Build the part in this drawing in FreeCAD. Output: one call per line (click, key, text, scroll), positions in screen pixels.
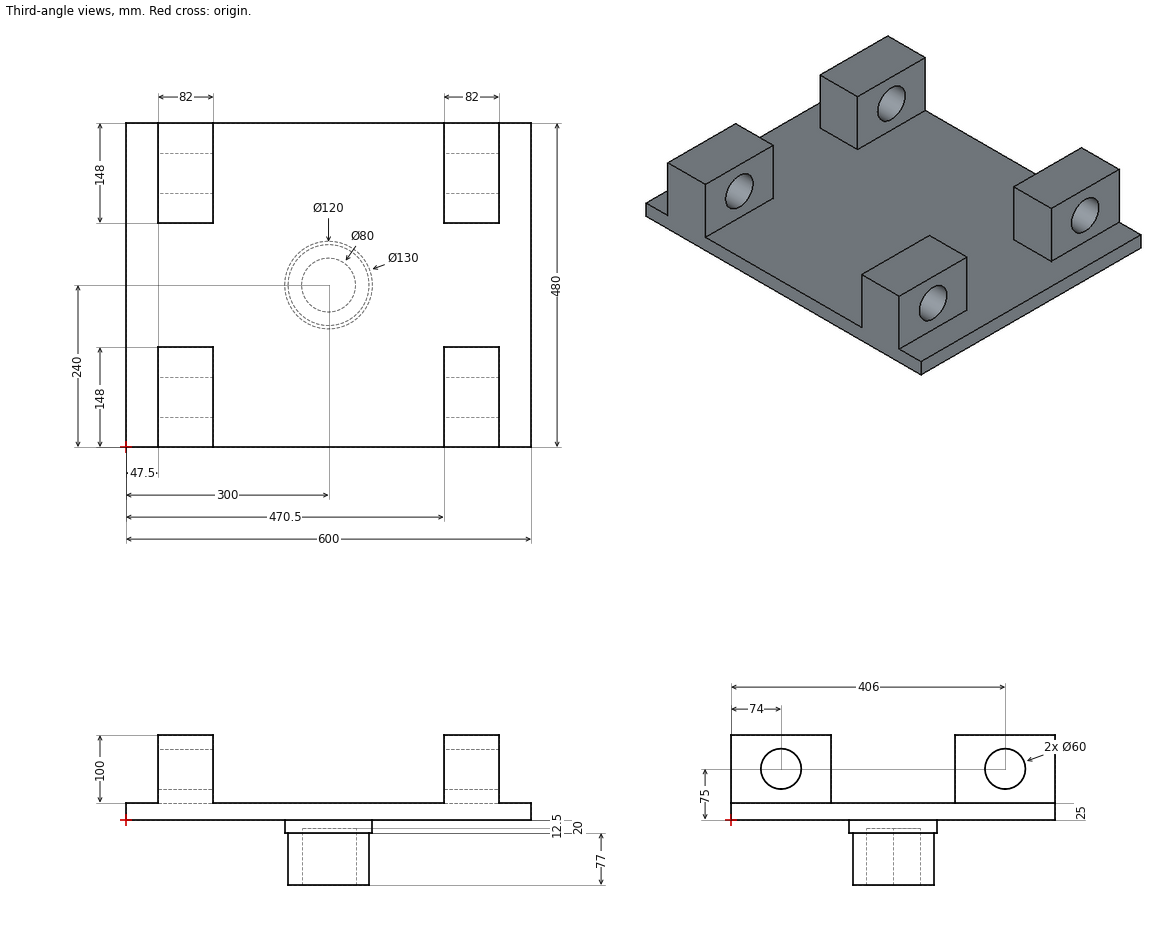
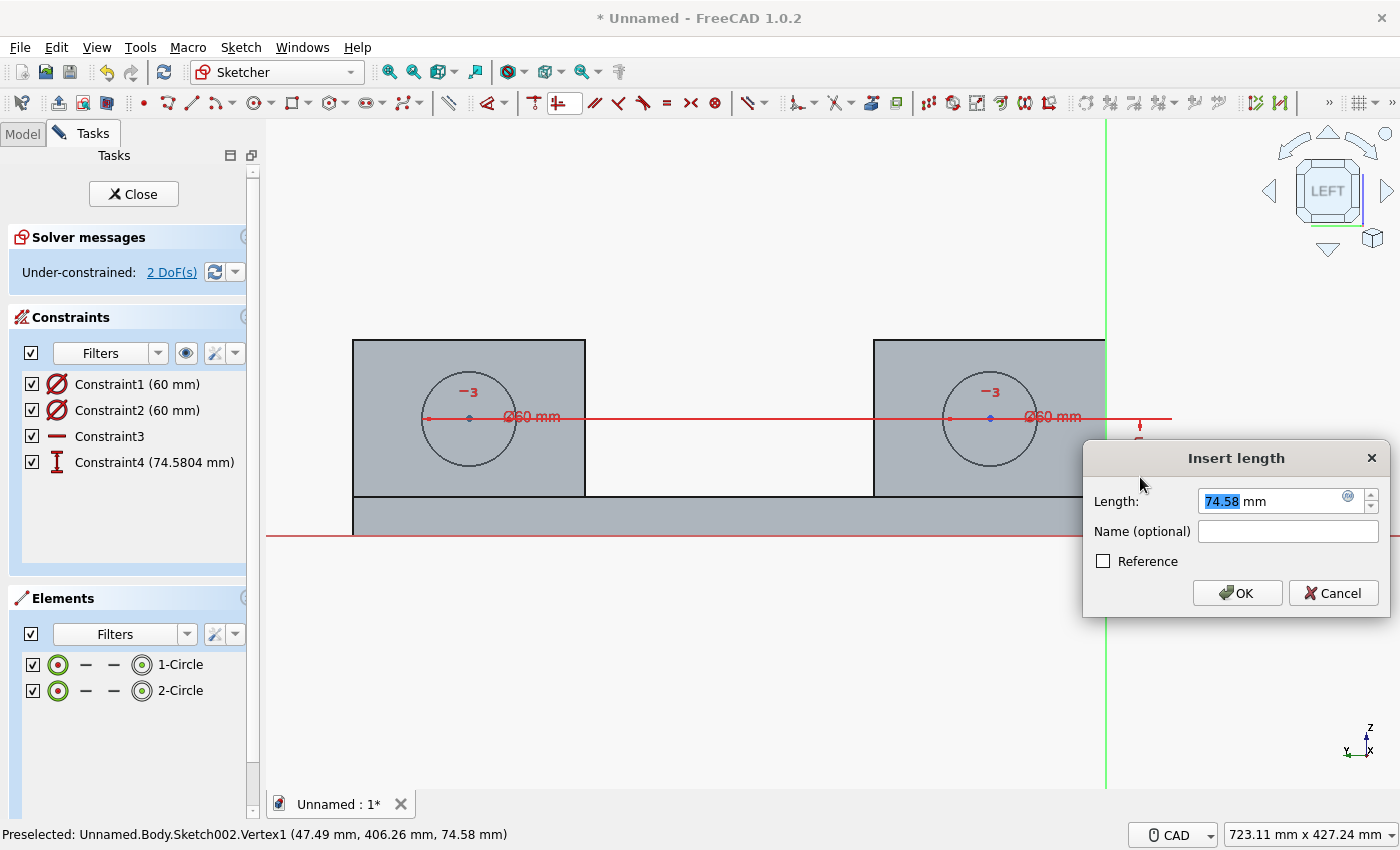
text(75)
key(Return)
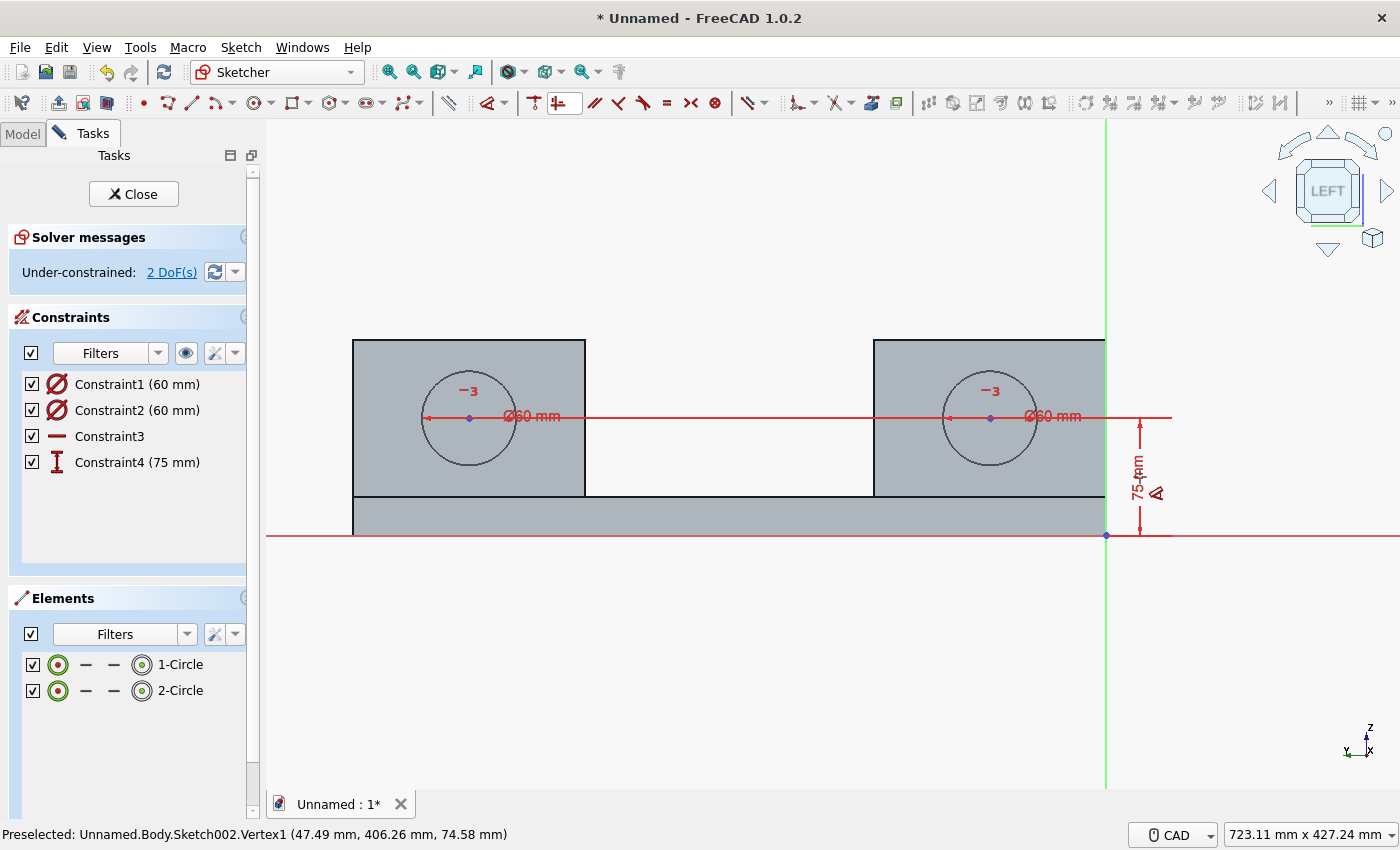
click(990, 418)
click(1048, 570)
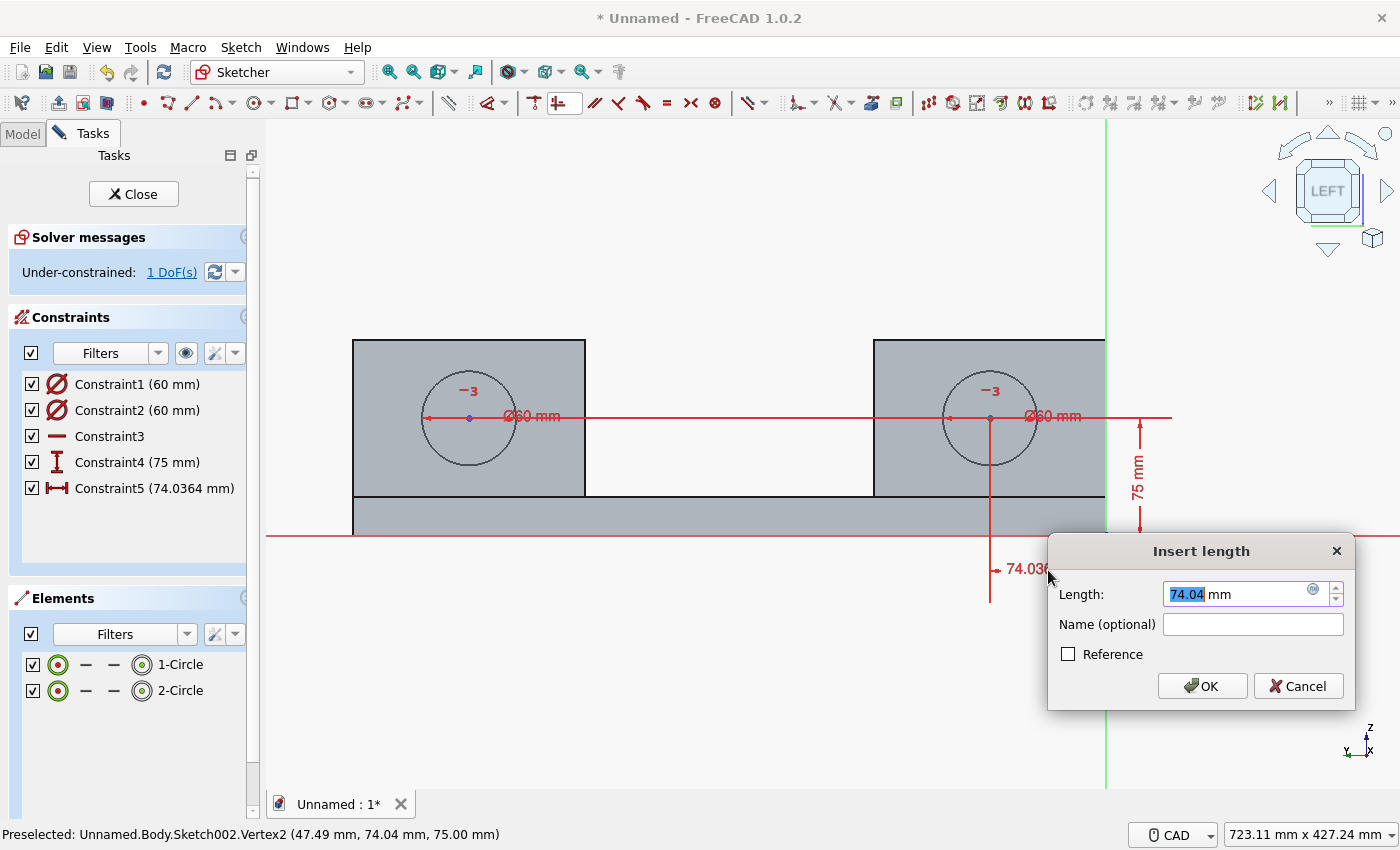
text(74)
key(Return)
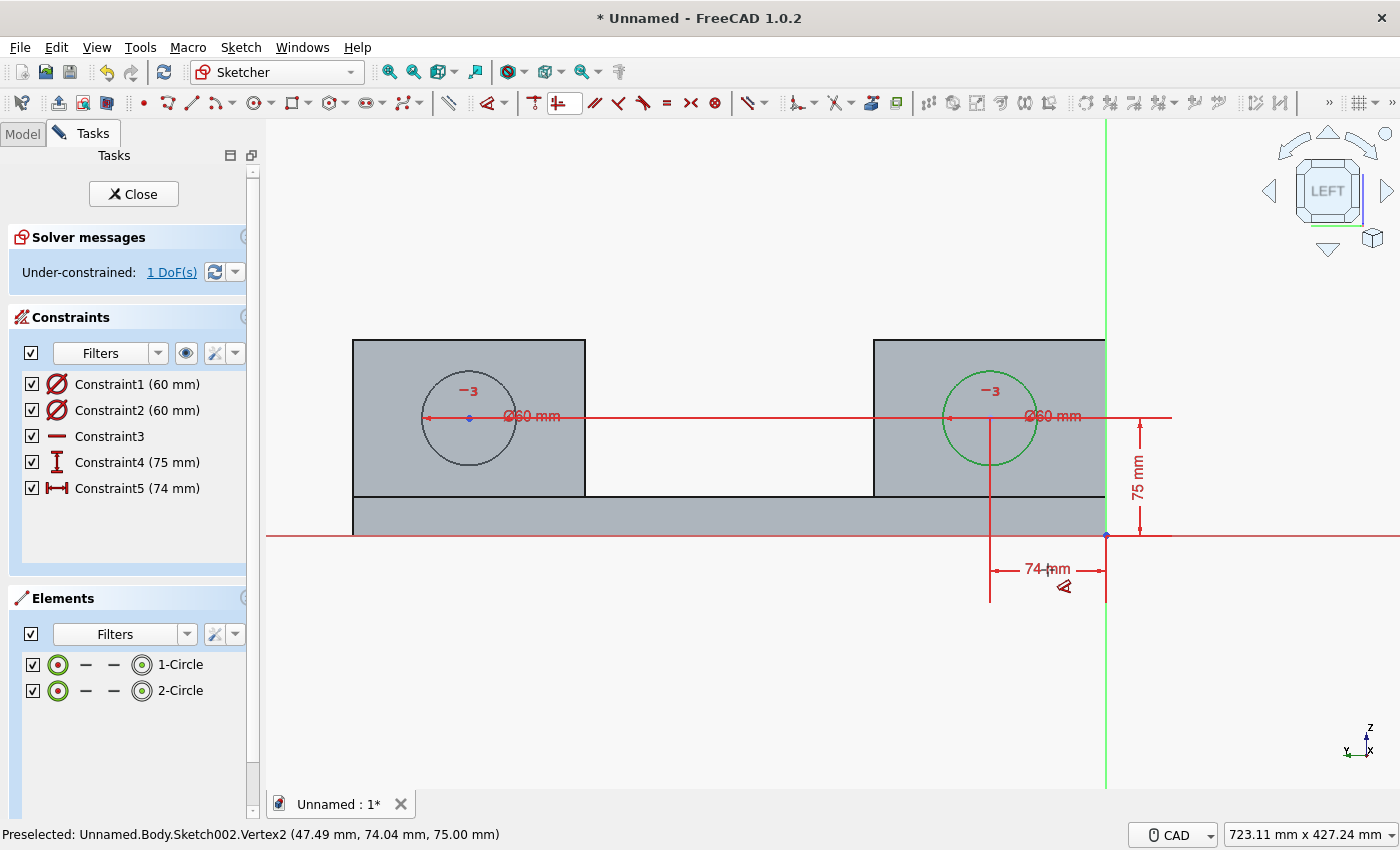
click(469, 418)
click(788, 570)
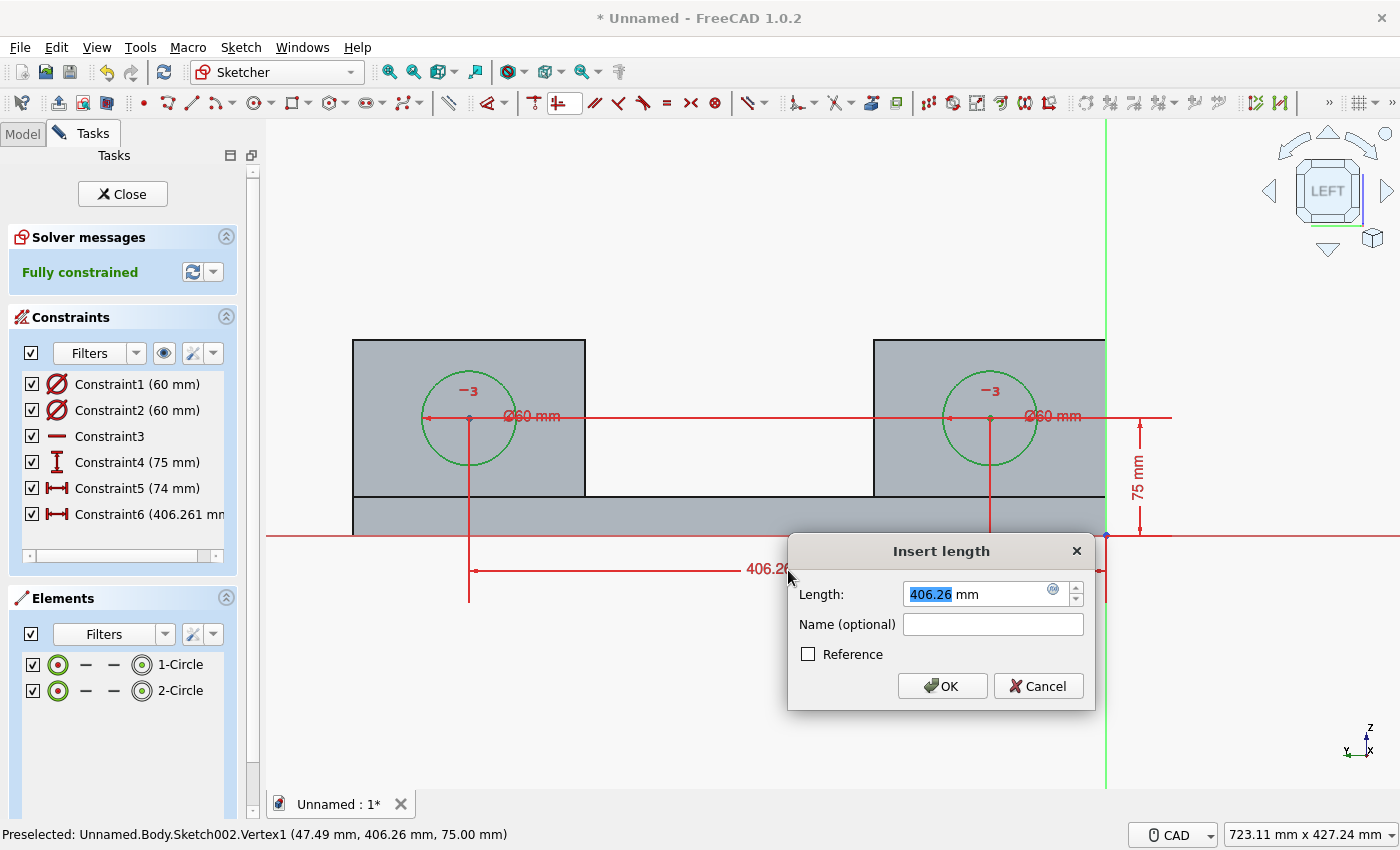
text(406)
key(Return)
key(Escape)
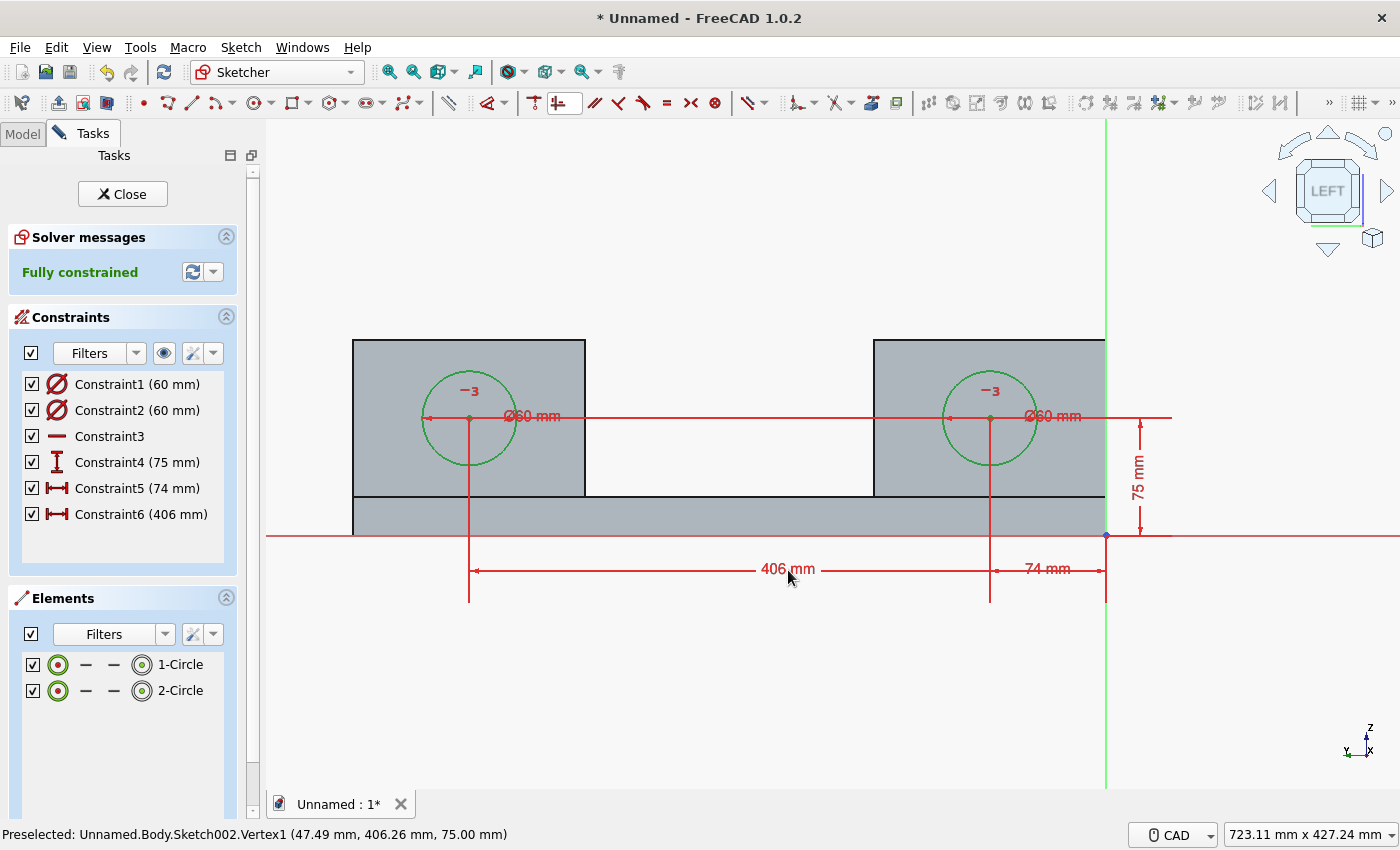
click(123, 194)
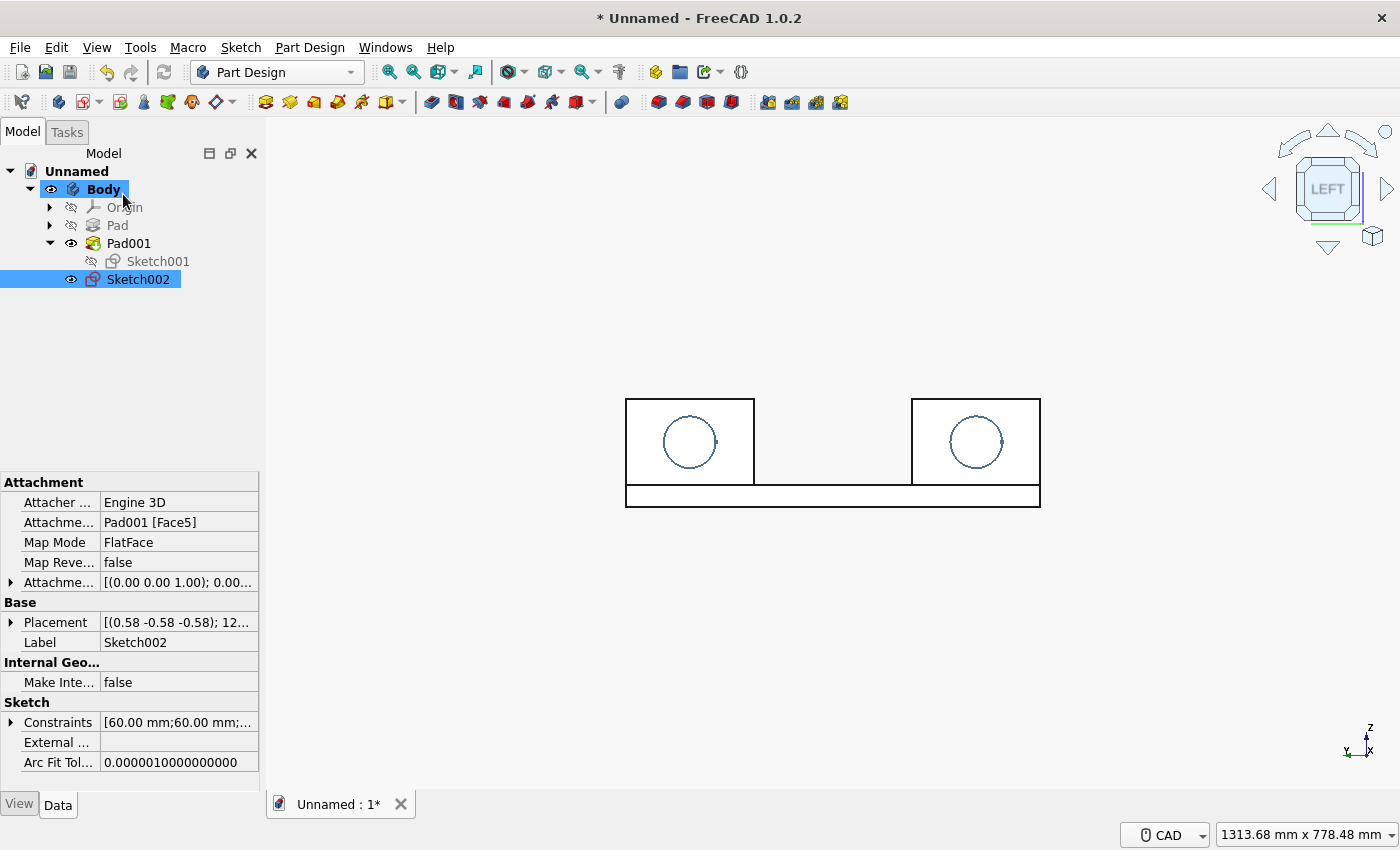
click(432, 102)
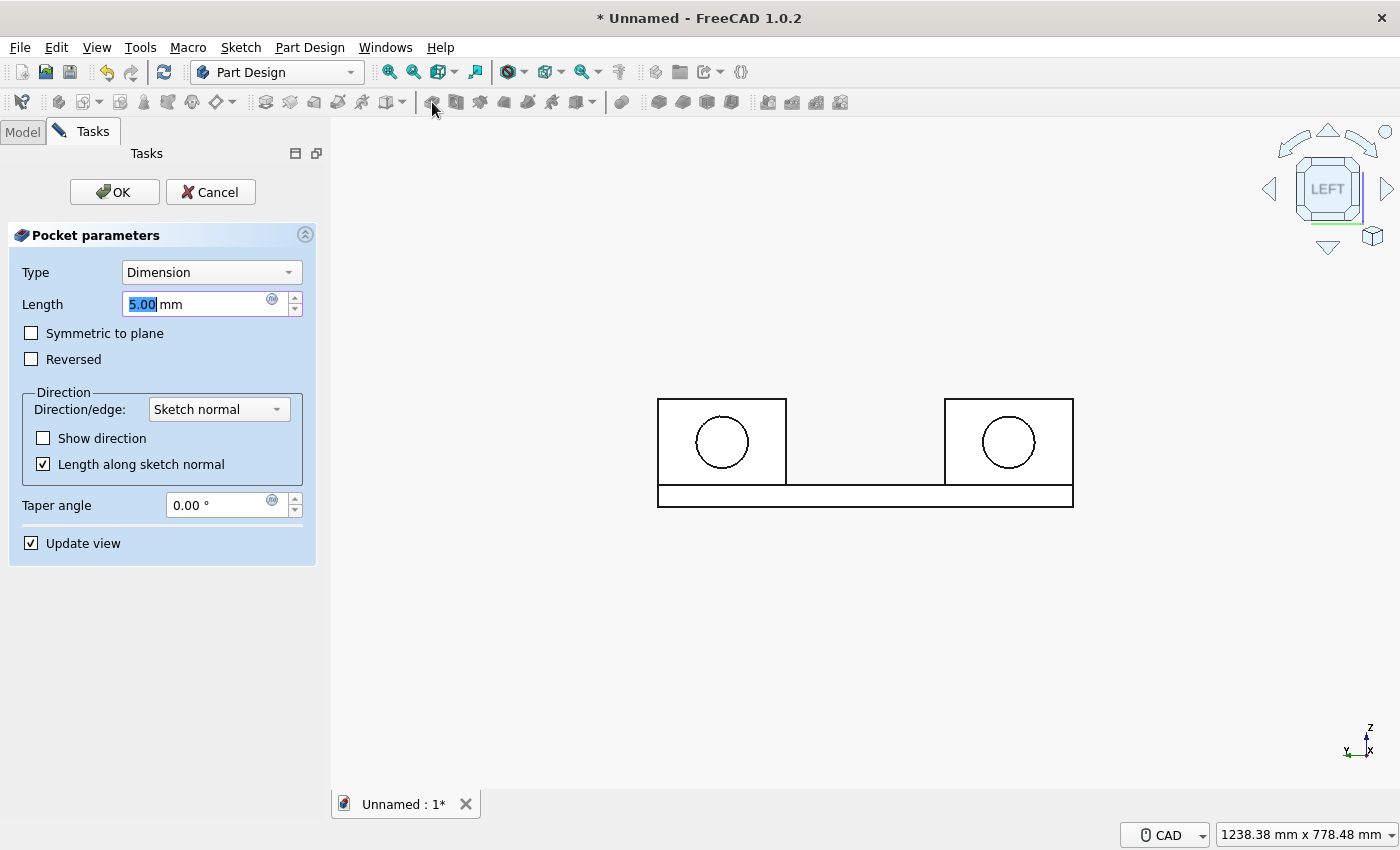
click(212, 272)